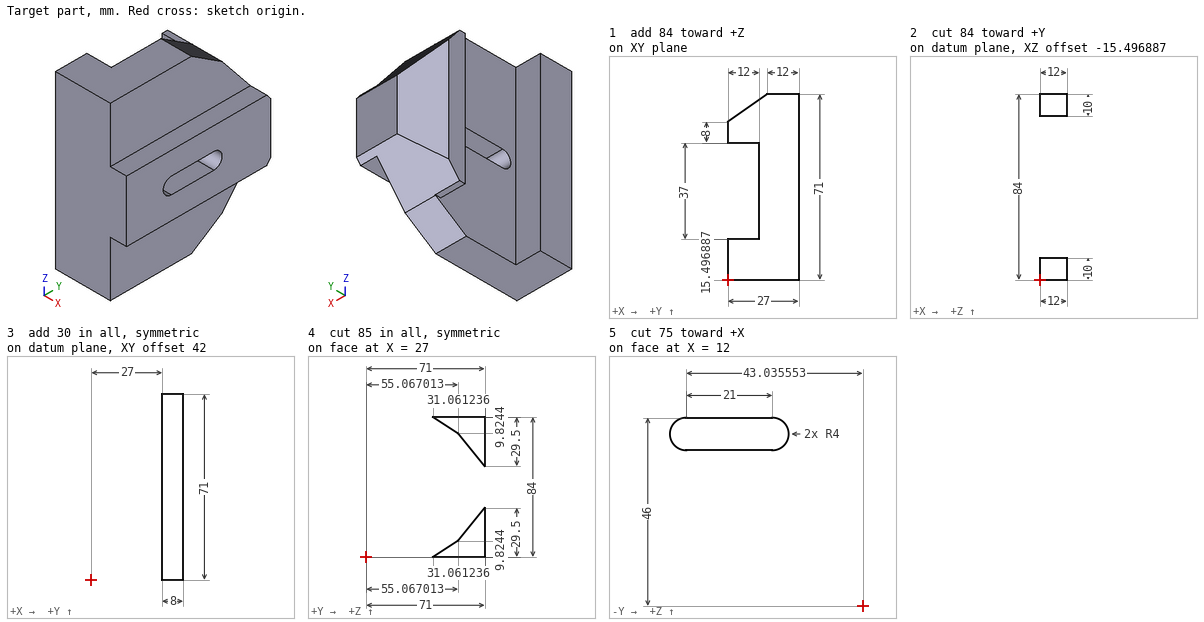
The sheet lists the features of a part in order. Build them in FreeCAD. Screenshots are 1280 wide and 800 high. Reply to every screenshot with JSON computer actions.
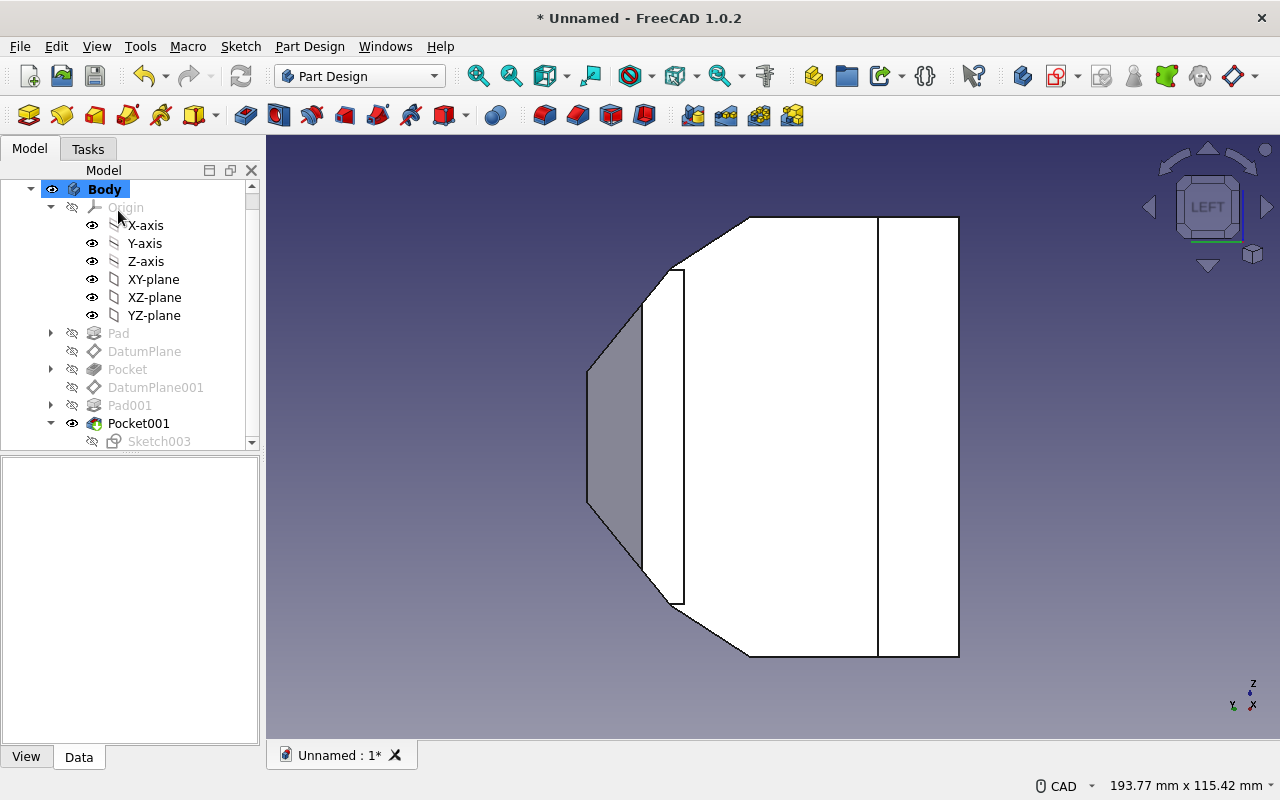
{"action": "left_click", "coordinate": [774, 310]}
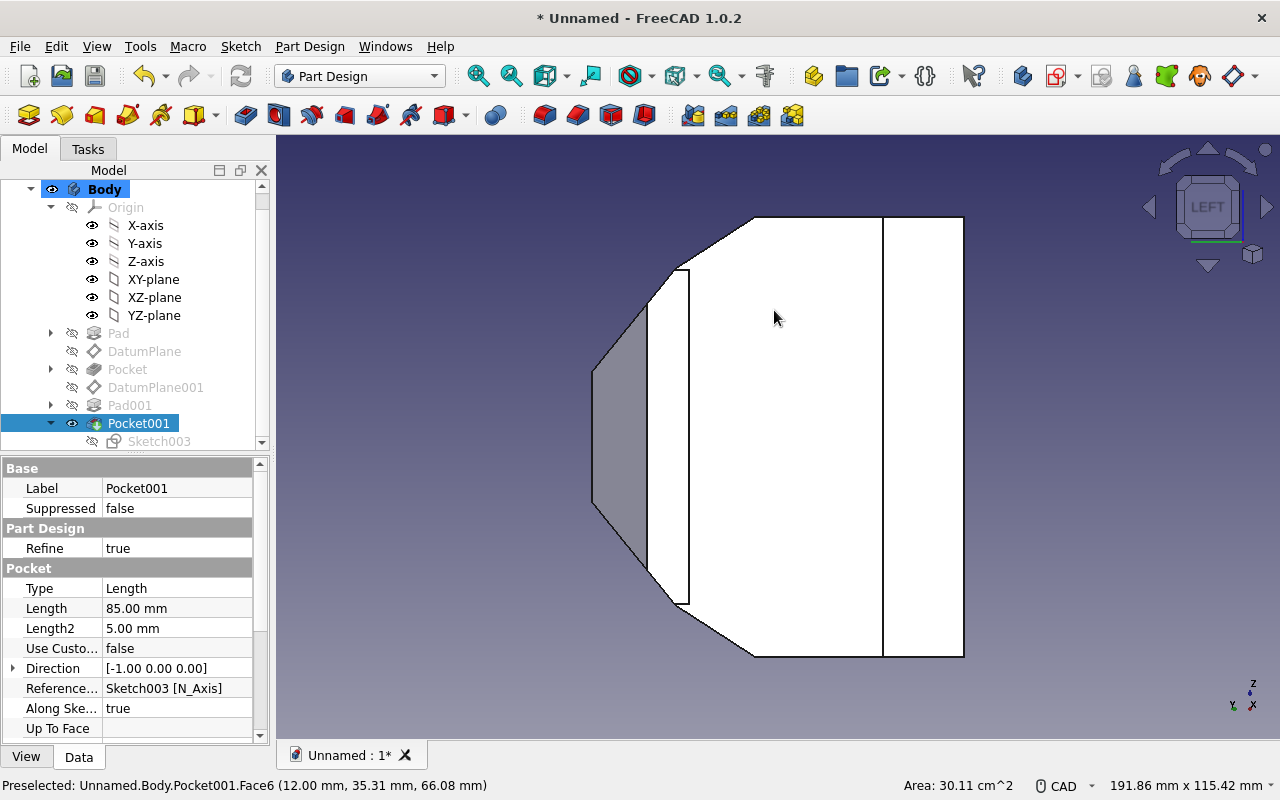
{"action": "left_click", "coordinate": [1056, 76]}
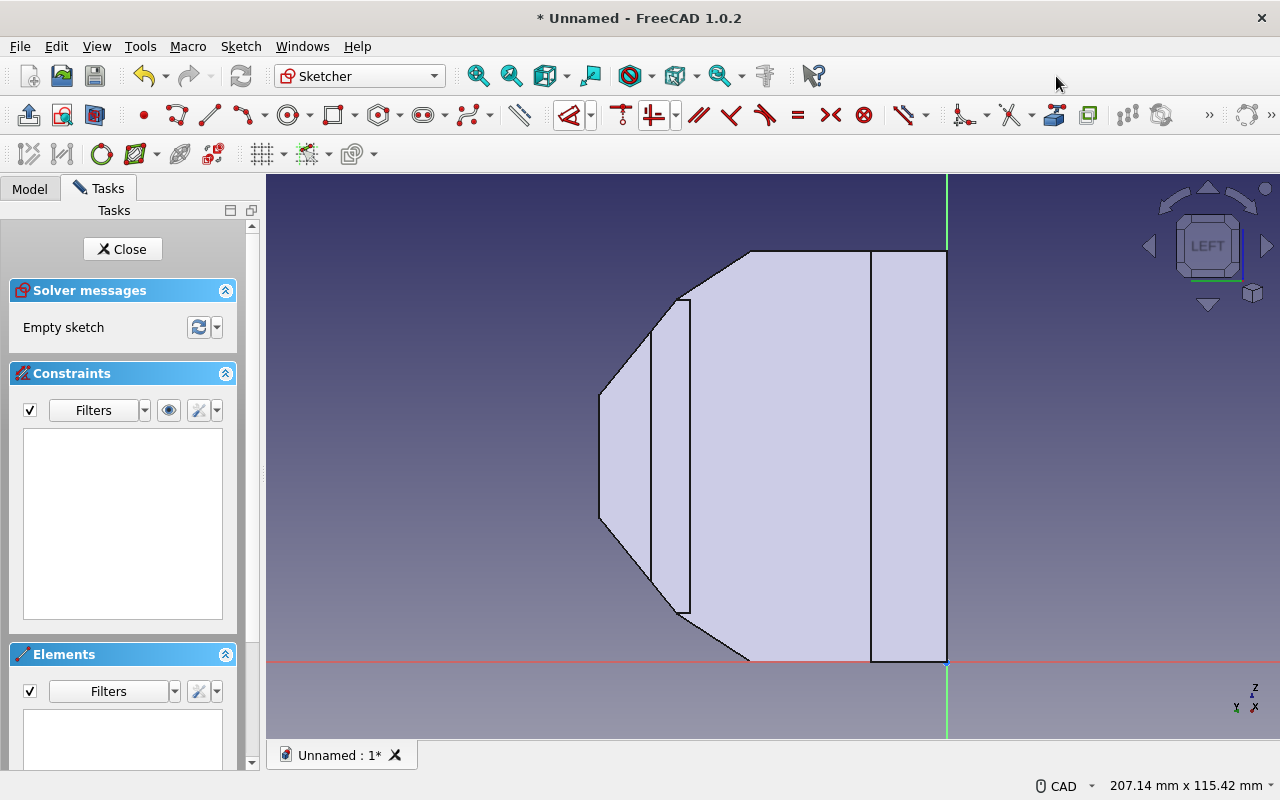
{"action": "scroll", "coordinate": [1090, 711], "scroll_direction": "up", "scroll_amount": 2}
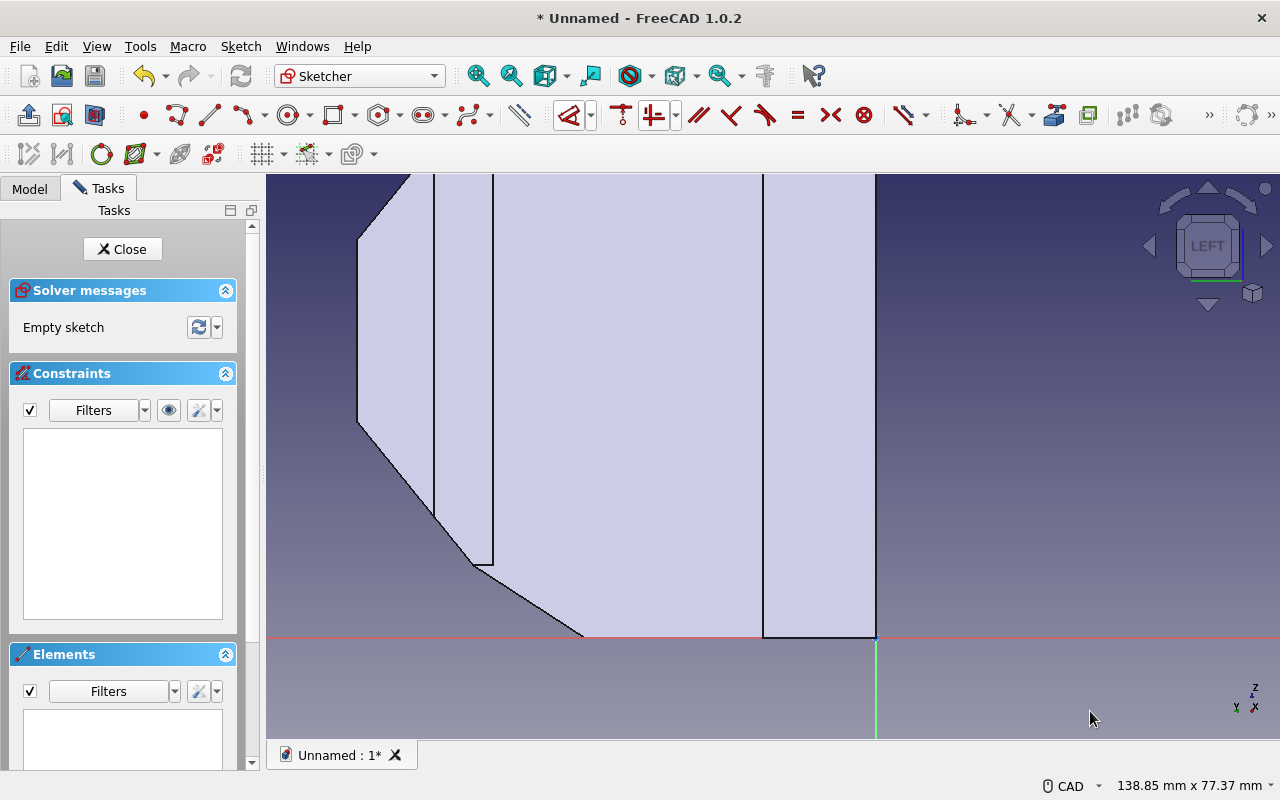
{"action": "left_click", "coordinate": [422, 116]}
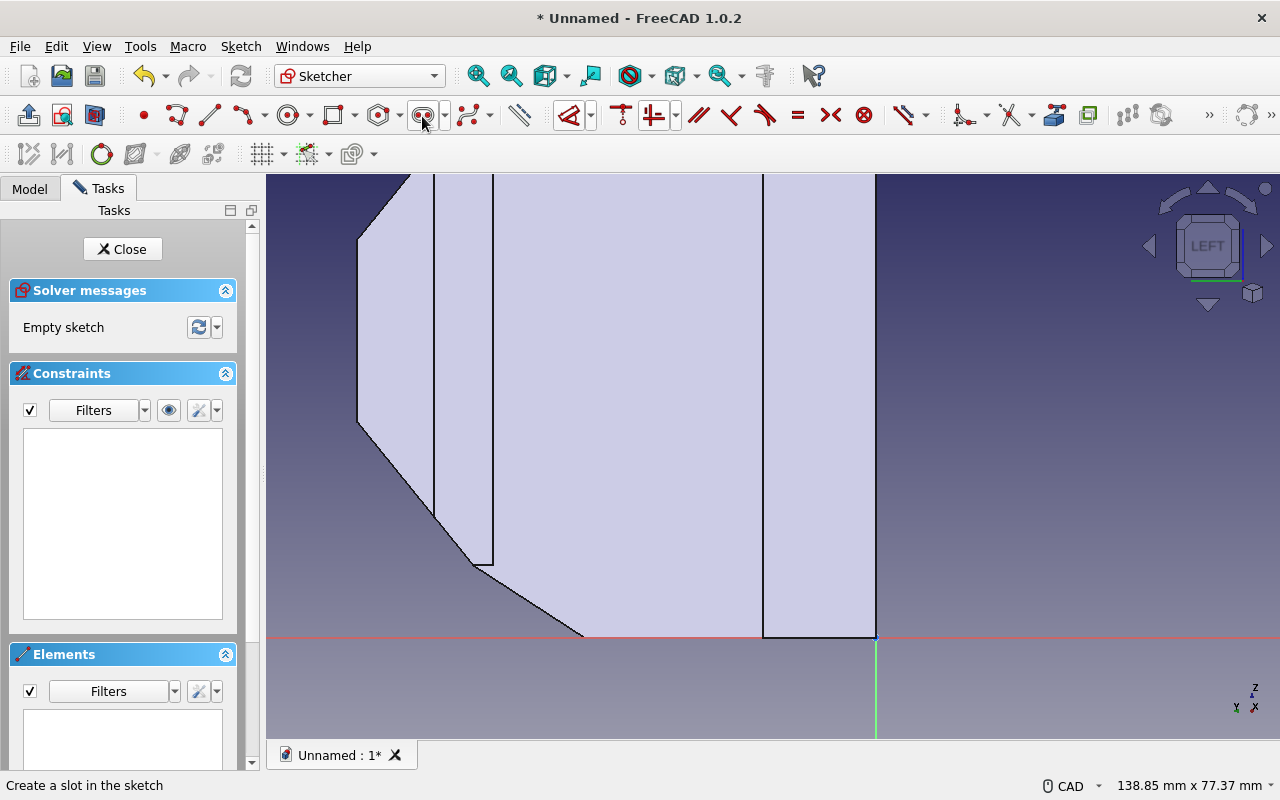
{"action": "left_click", "coordinate": [562, 331]}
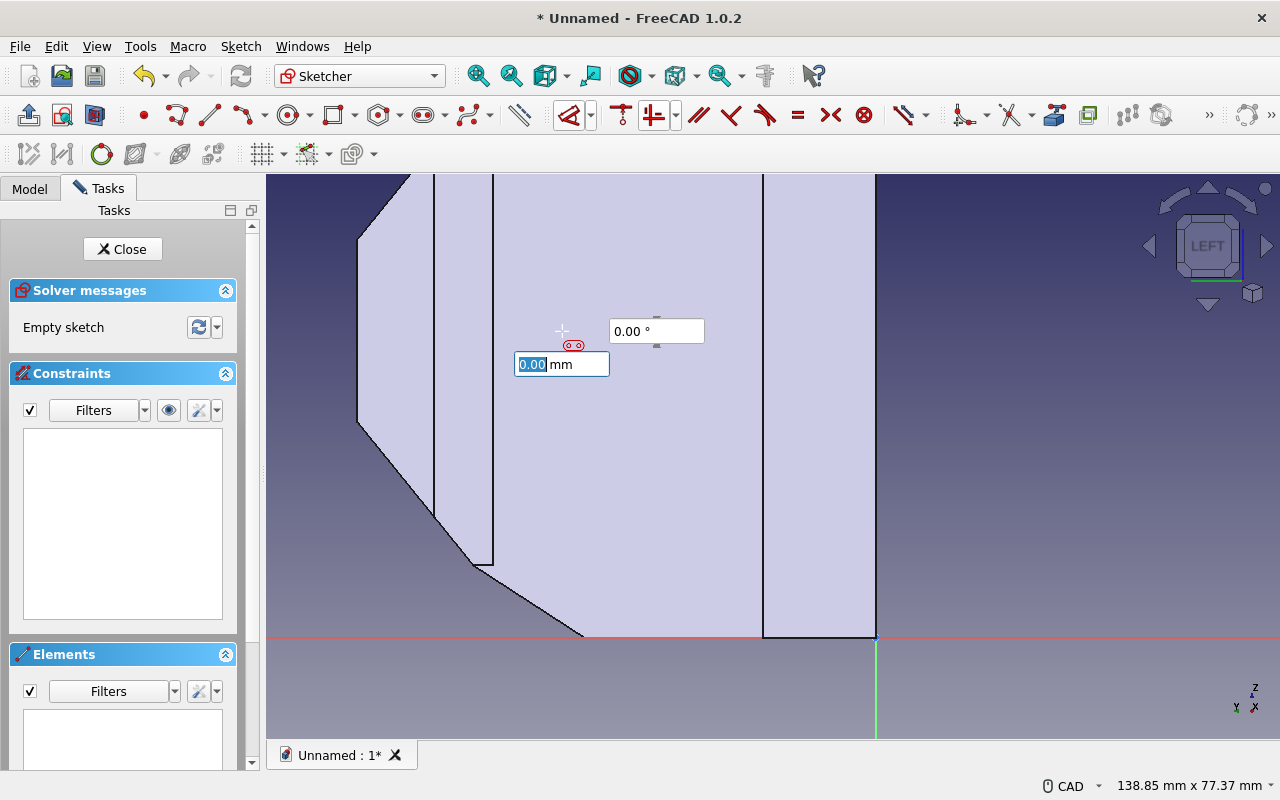
{"action": "left_click", "coordinate": [715, 331]}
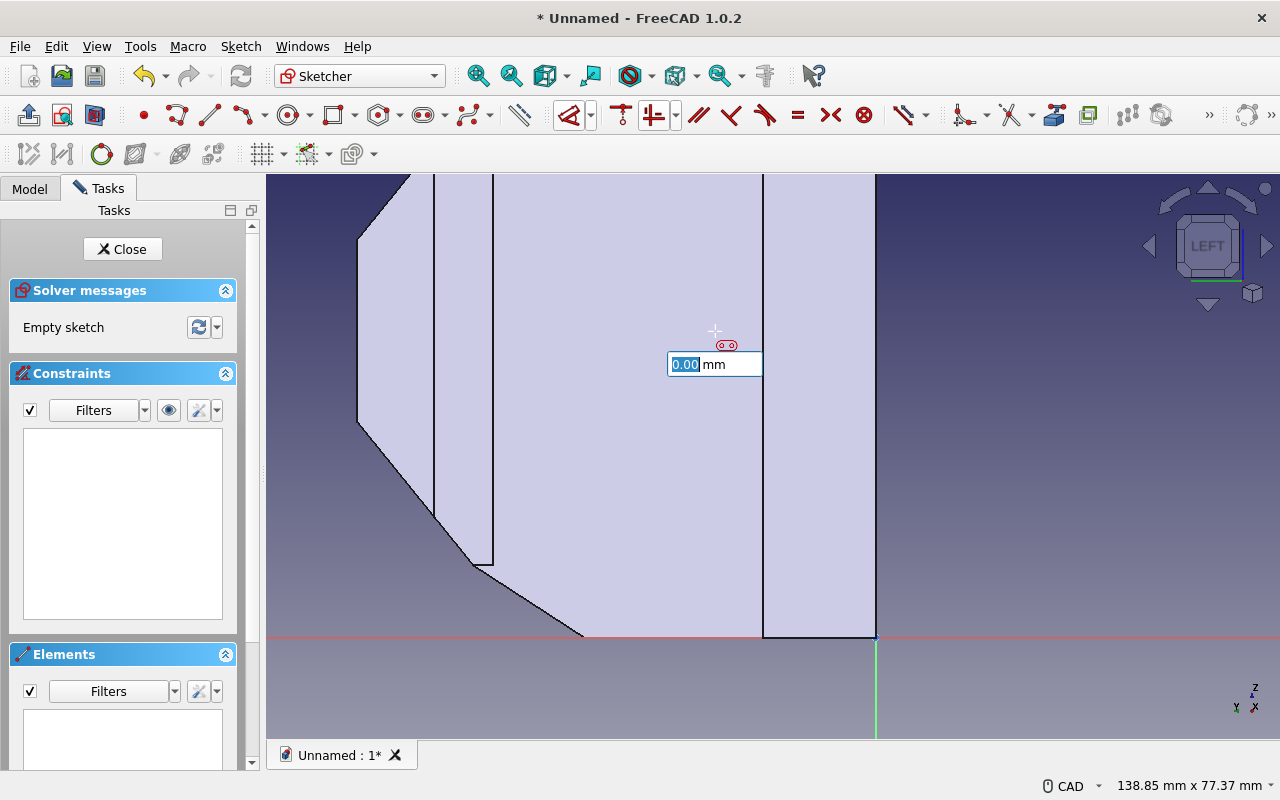
{"action": "left_click", "coordinate": [638, 302]}
{"action": "key", "text": "Escape"}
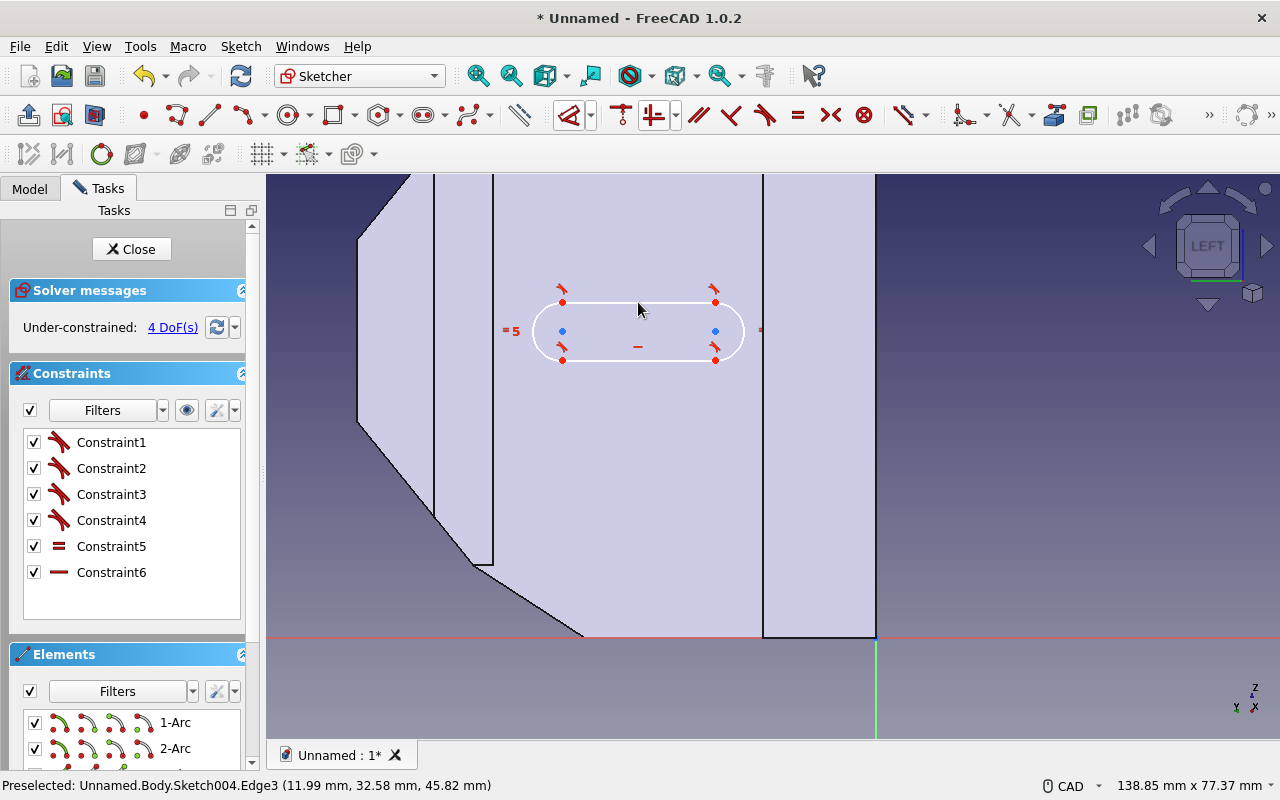
{"action": "scroll", "coordinate": [539, 315], "scroll_direction": "up", "scroll_amount": 2}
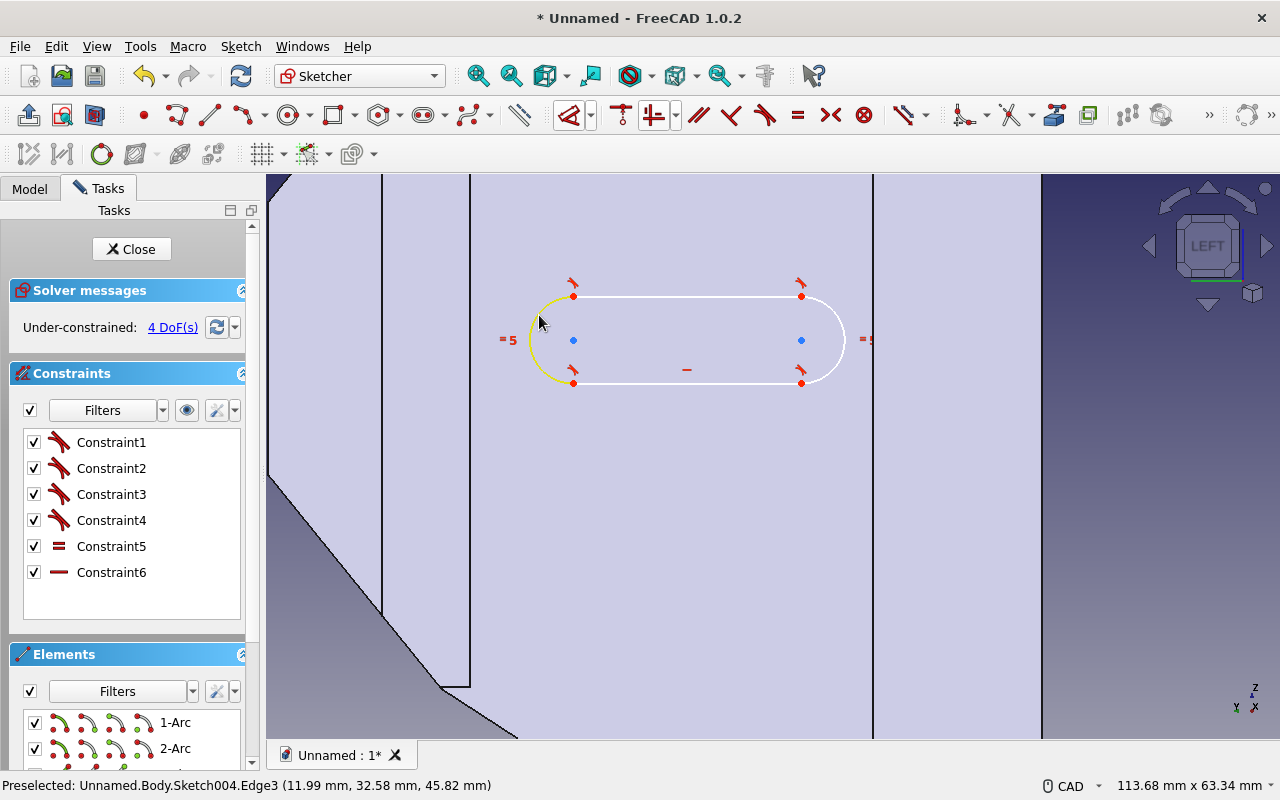
{"action": "left_click", "coordinate": [538, 315]}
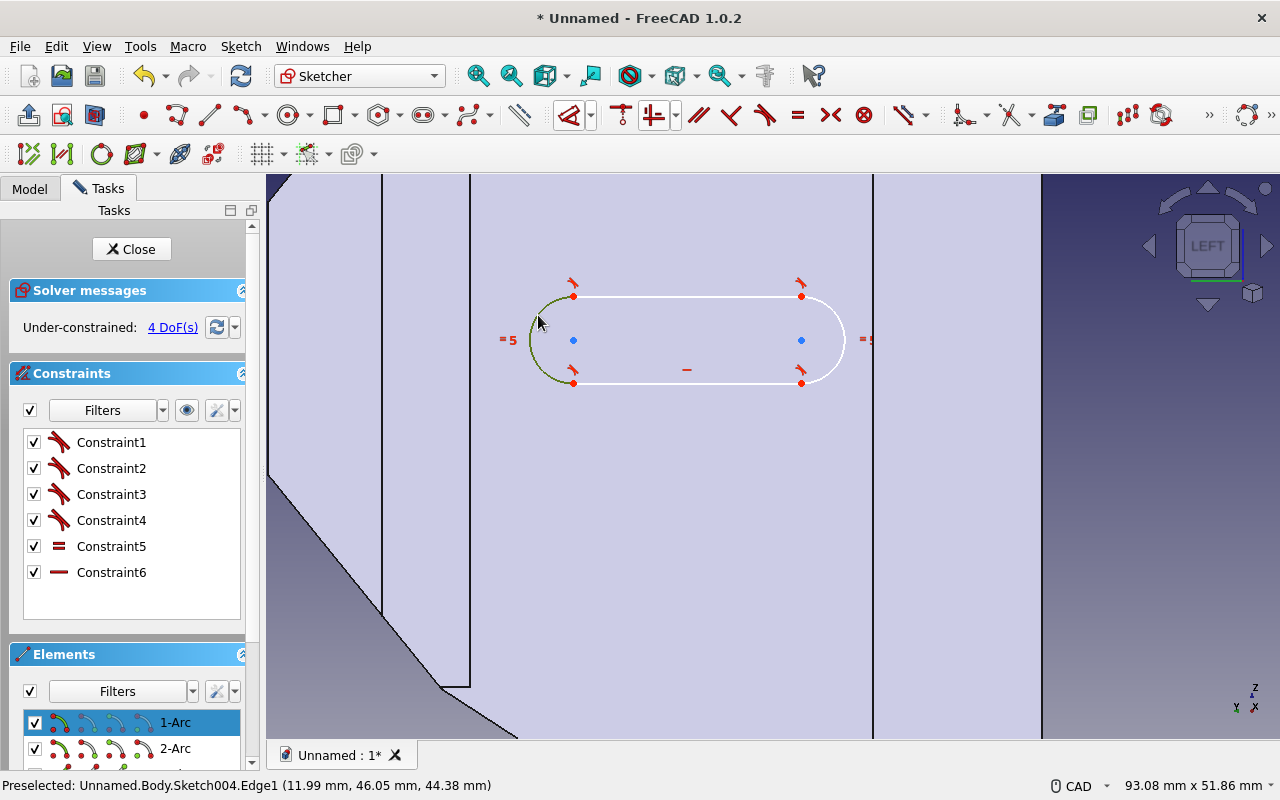
{"action": "key", "text": "k r"}